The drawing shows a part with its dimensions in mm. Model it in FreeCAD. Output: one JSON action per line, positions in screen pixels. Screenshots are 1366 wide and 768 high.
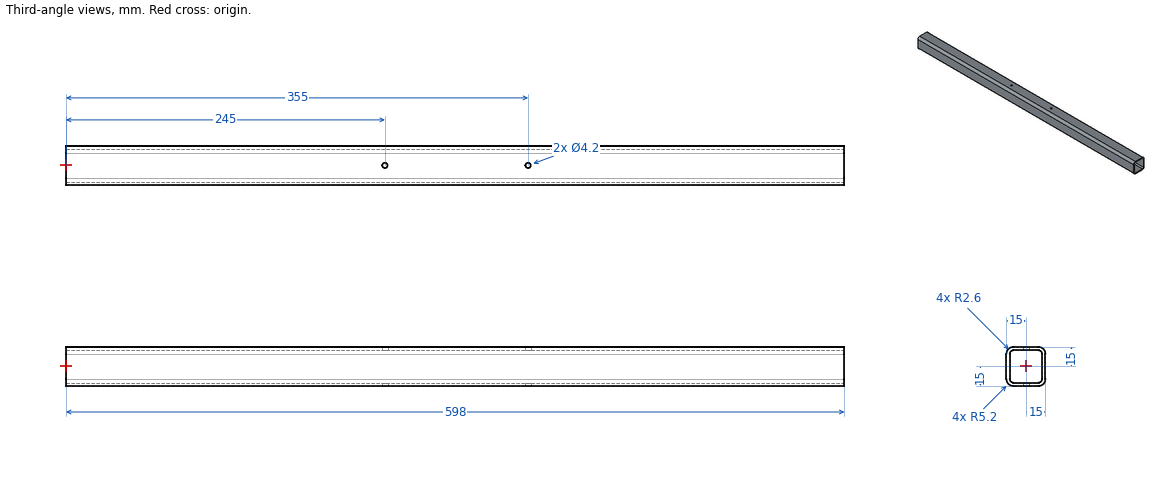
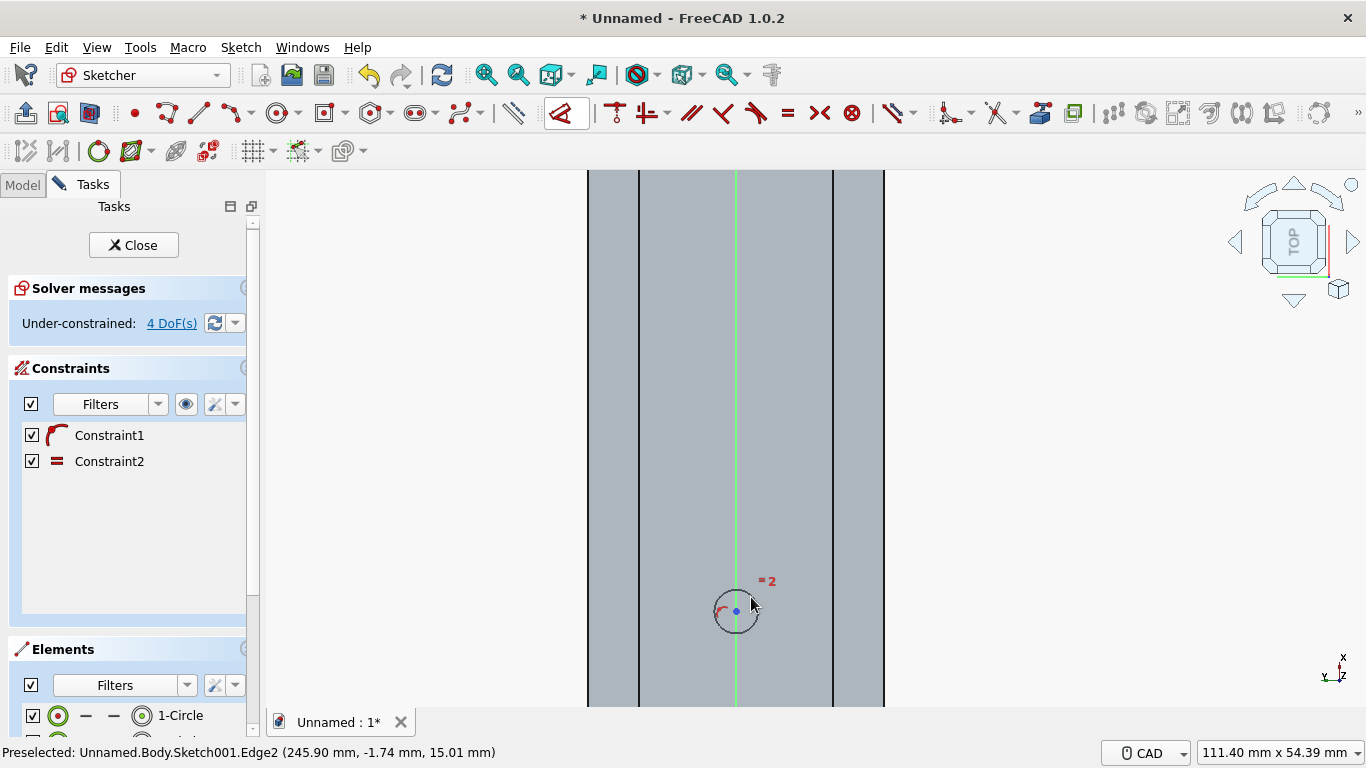
{"action": "scroll", "coordinate": [752, 599], "scroll_direction": "down", "scroll_amount": 6}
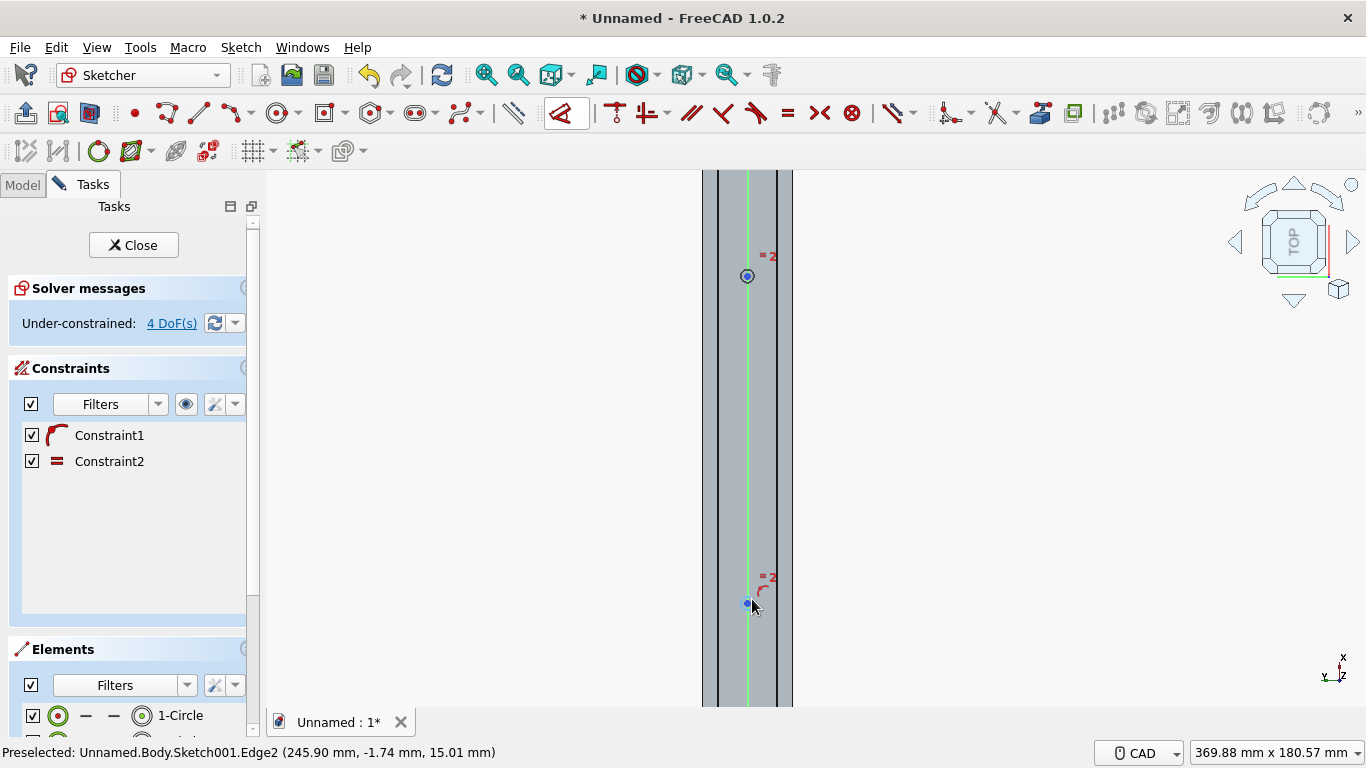
{"action": "left_click", "coordinate": [747, 276]}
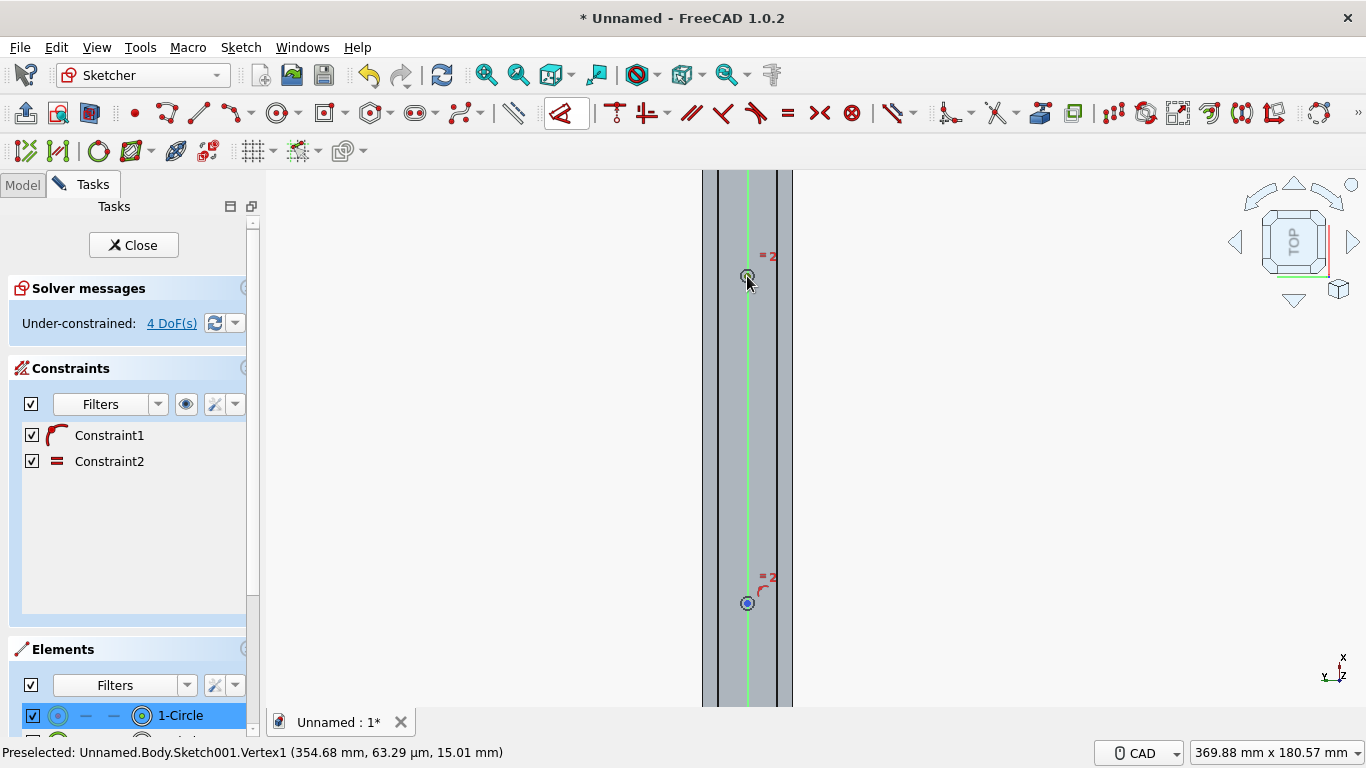
{"action": "left_click", "coordinate": [748, 645]}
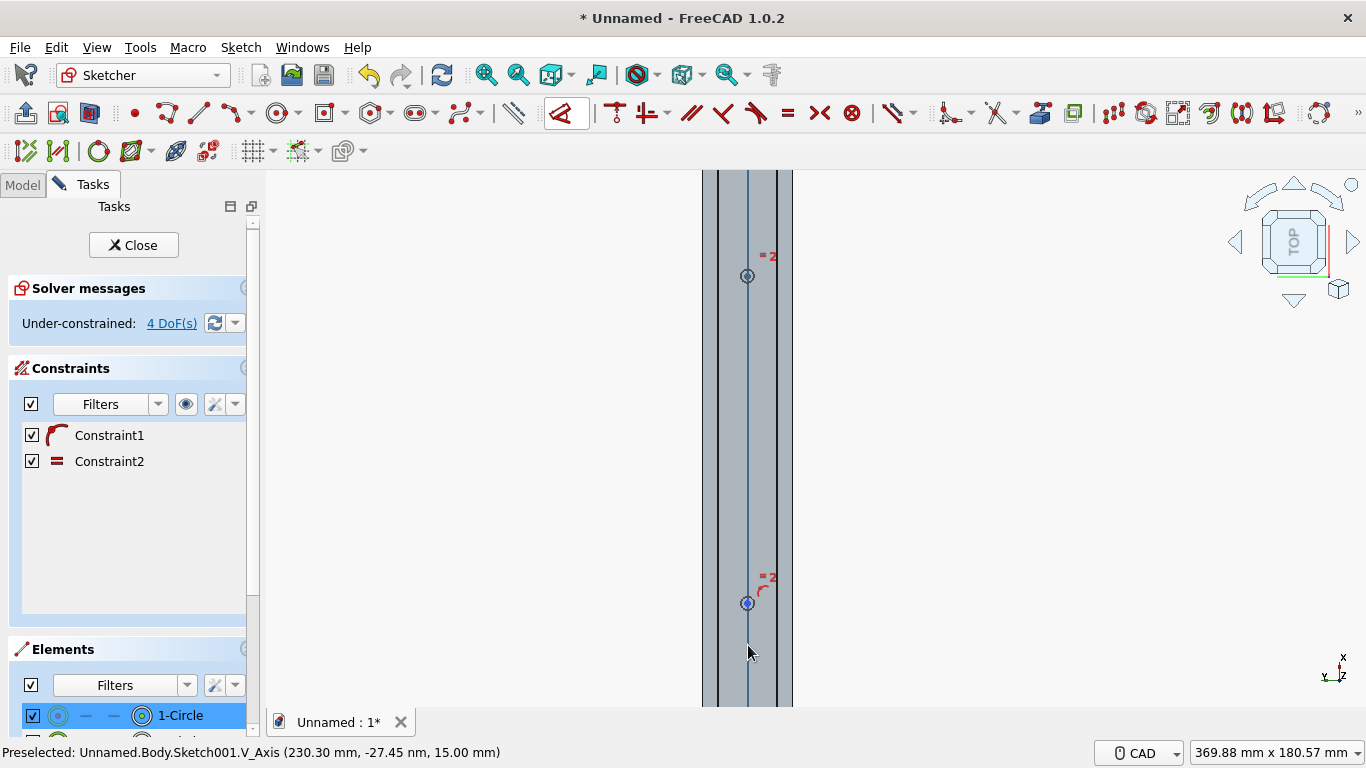
{"action": "key", "text": "c"}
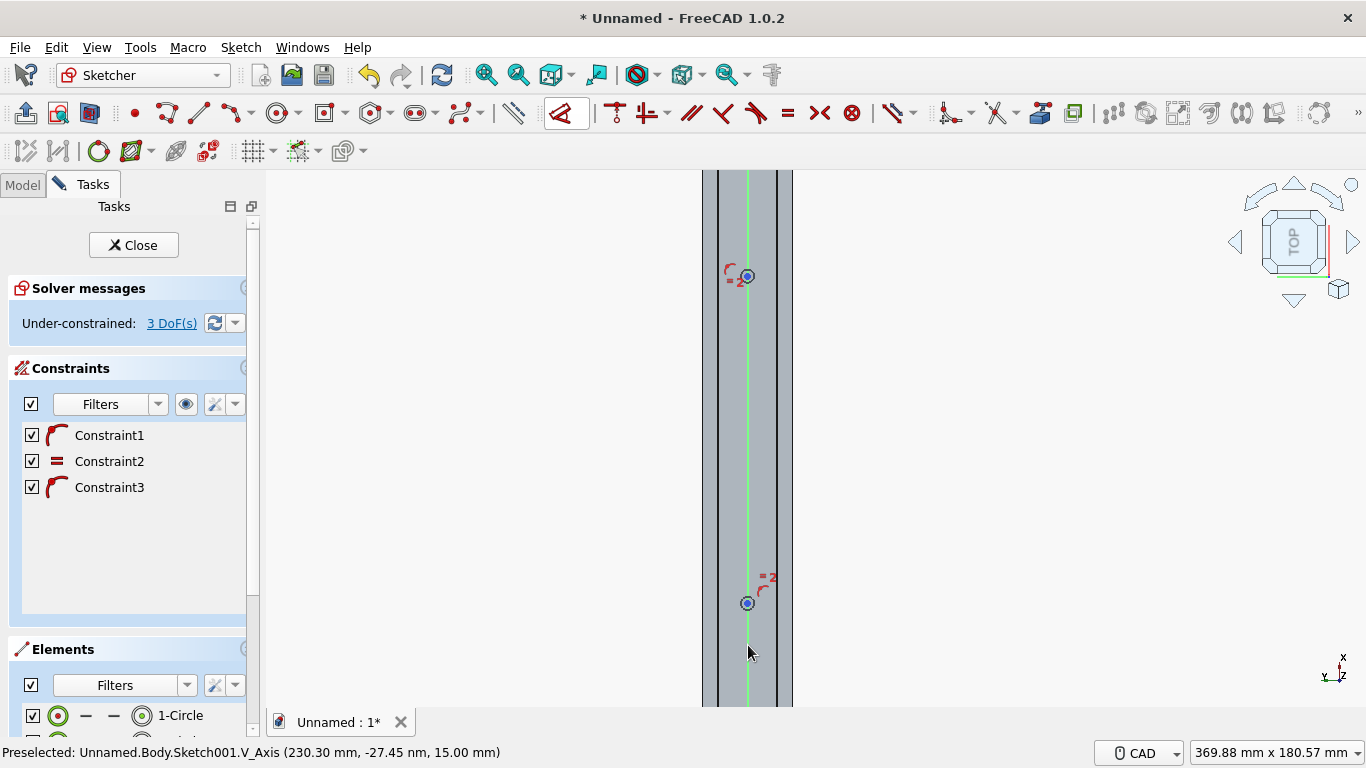
{"action": "key", "text": "d"}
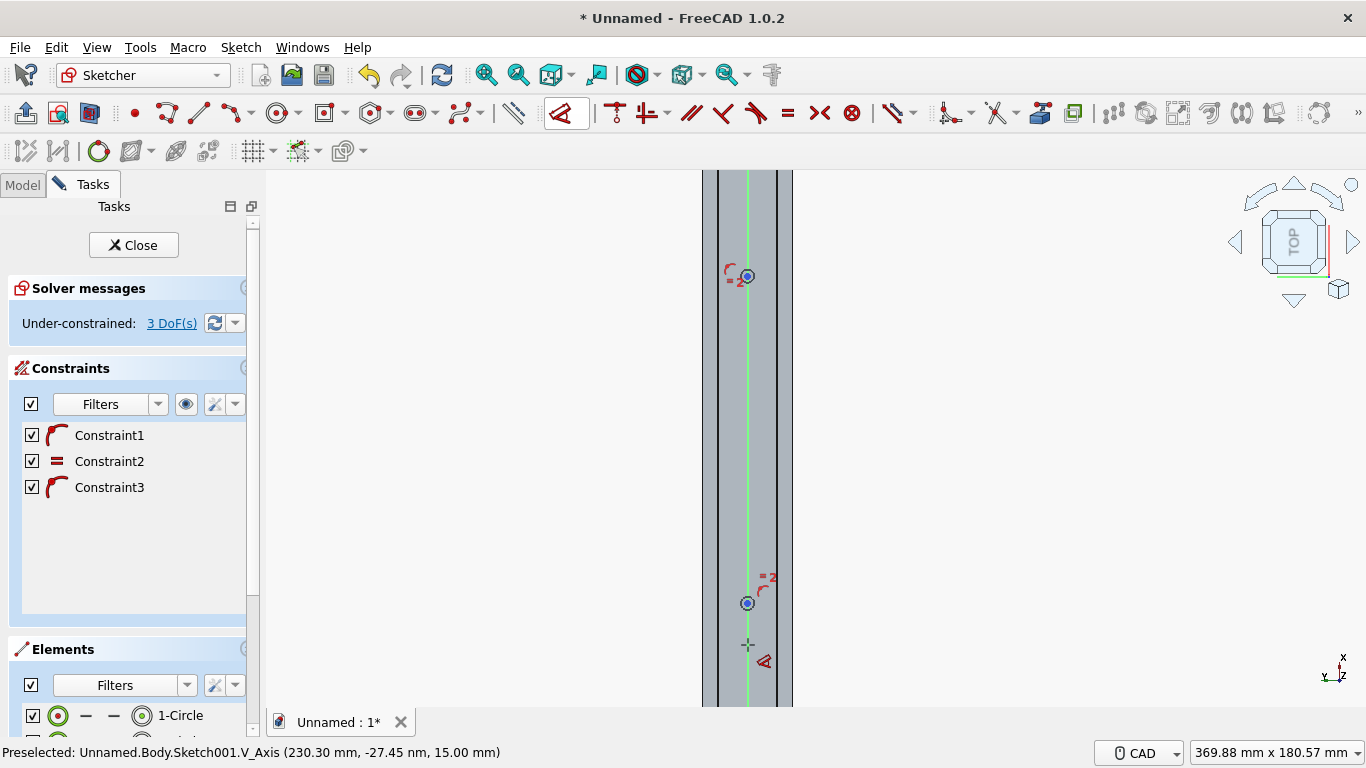
{"action": "scroll", "coordinate": [747, 283], "scroll_direction": "up", "scroll_amount": 6}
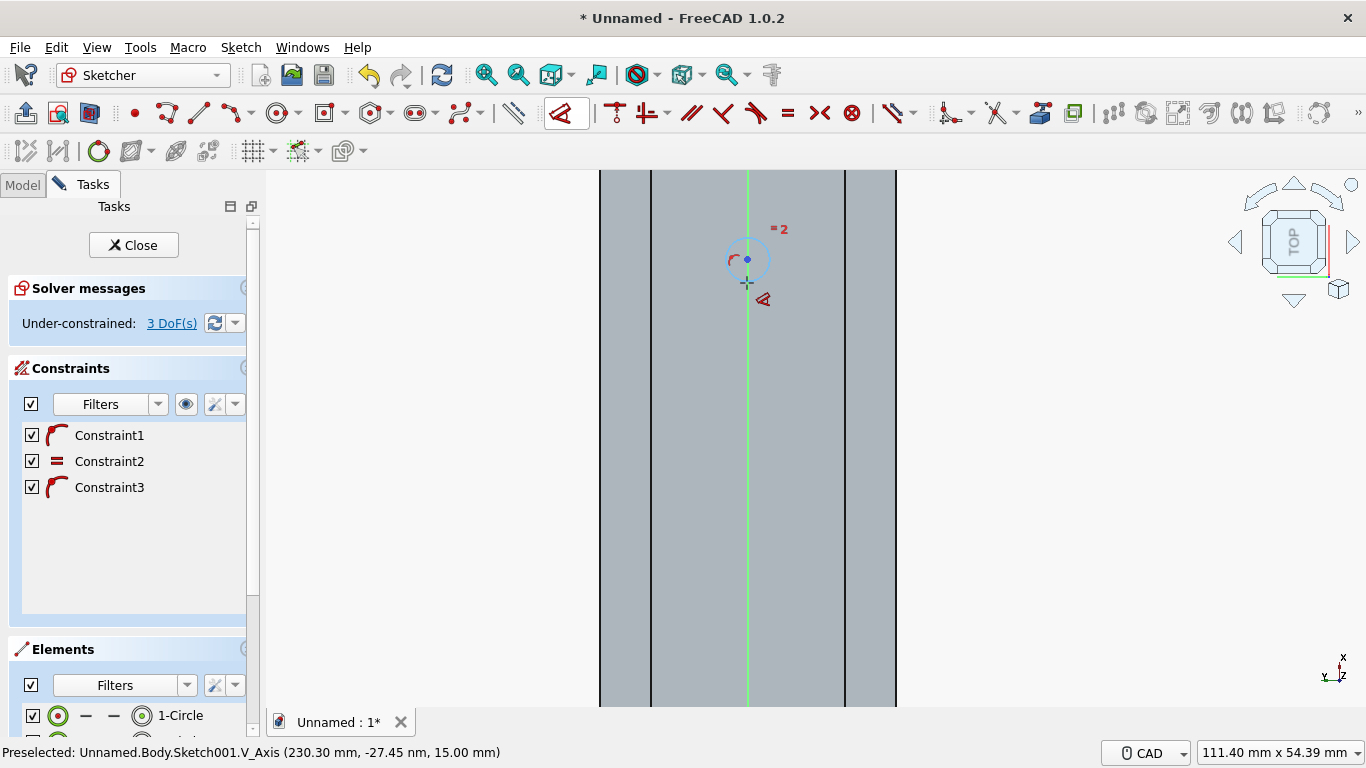
{"action": "left_click", "coordinate": [747, 281]}
{"action": "left_click", "coordinate": [720, 305]}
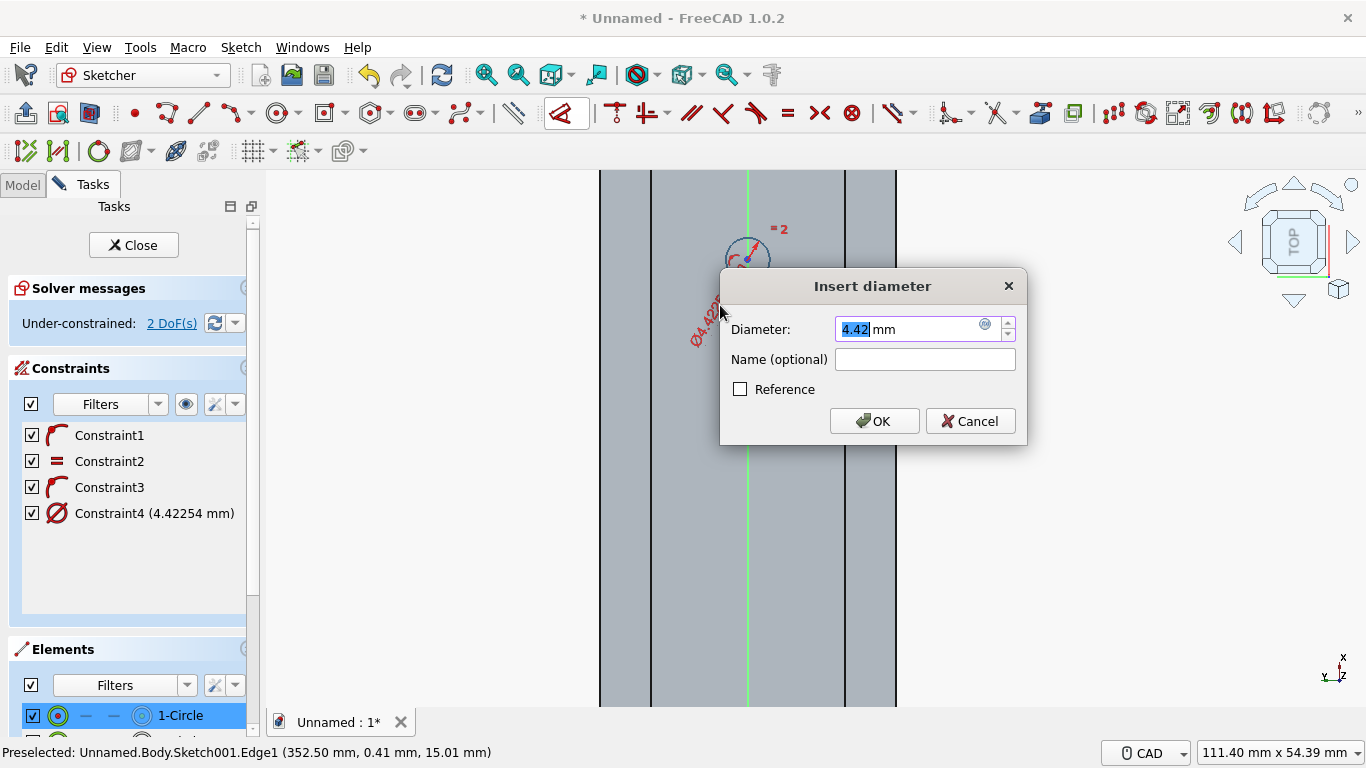
{"action": "type", "text": "4.2"}
{"action": "key", "text": "Return"}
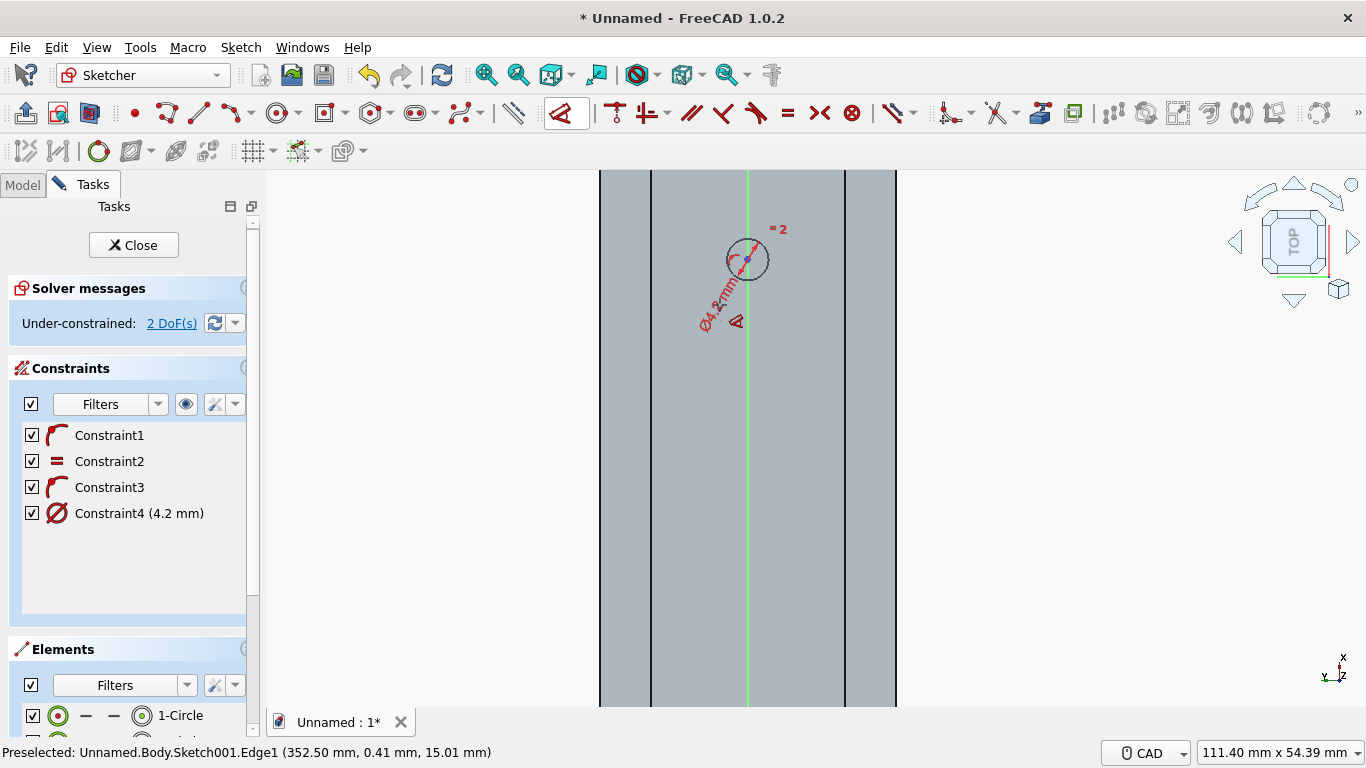
{"action": "left_click", "coordinate": [748, 260]}
{"action": "left_click", "coordinate": [782, 469]}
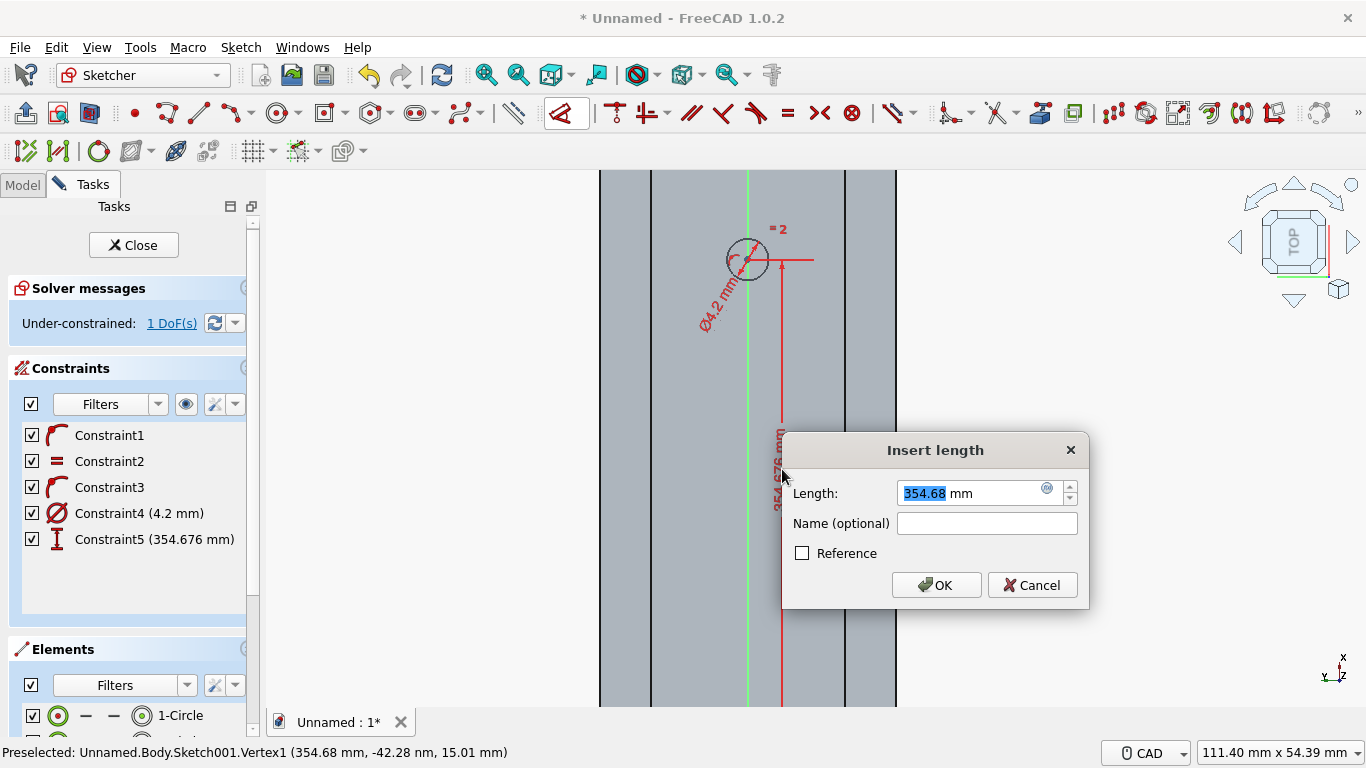
{"action": "type", "text": "355"}
{"action": "key", "text": "Return"}